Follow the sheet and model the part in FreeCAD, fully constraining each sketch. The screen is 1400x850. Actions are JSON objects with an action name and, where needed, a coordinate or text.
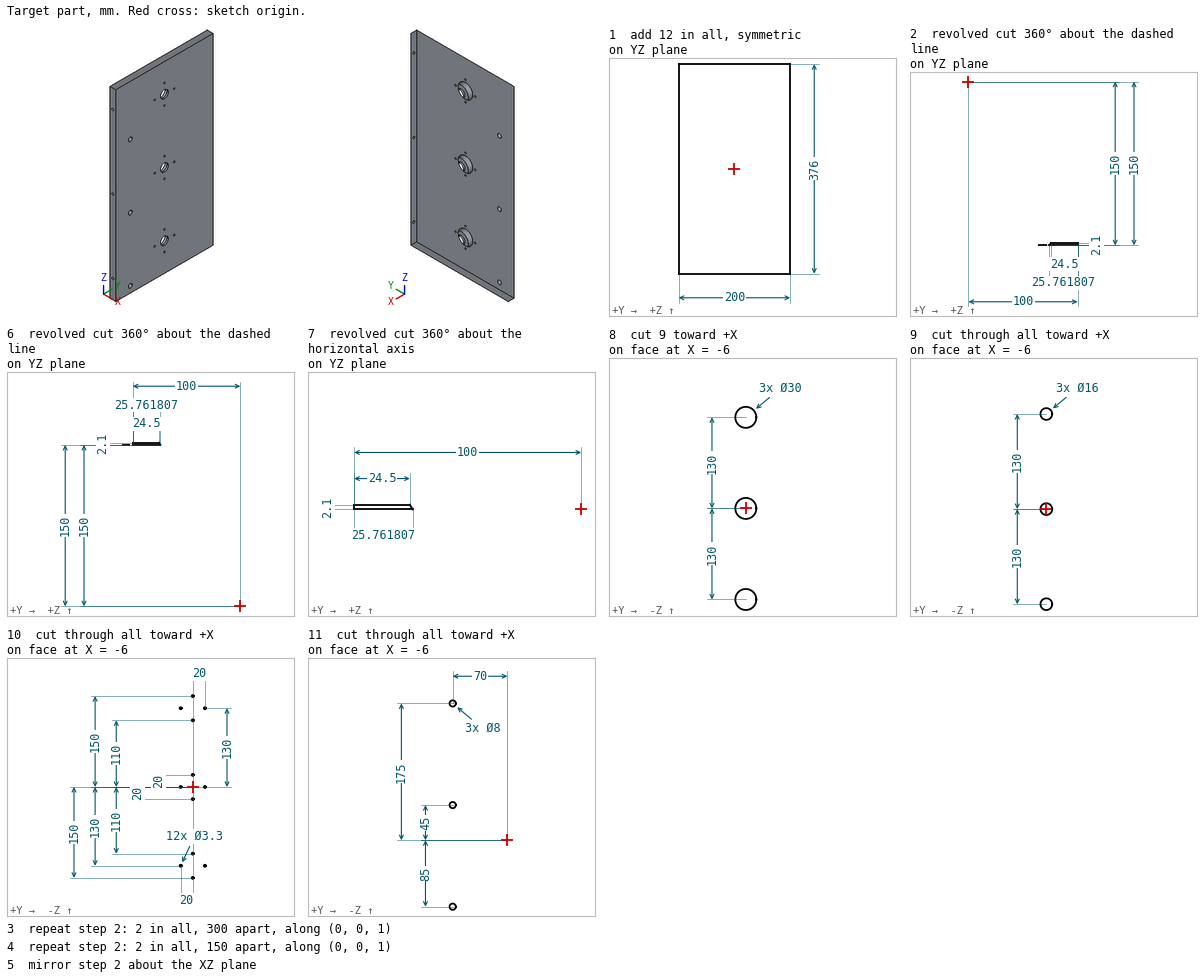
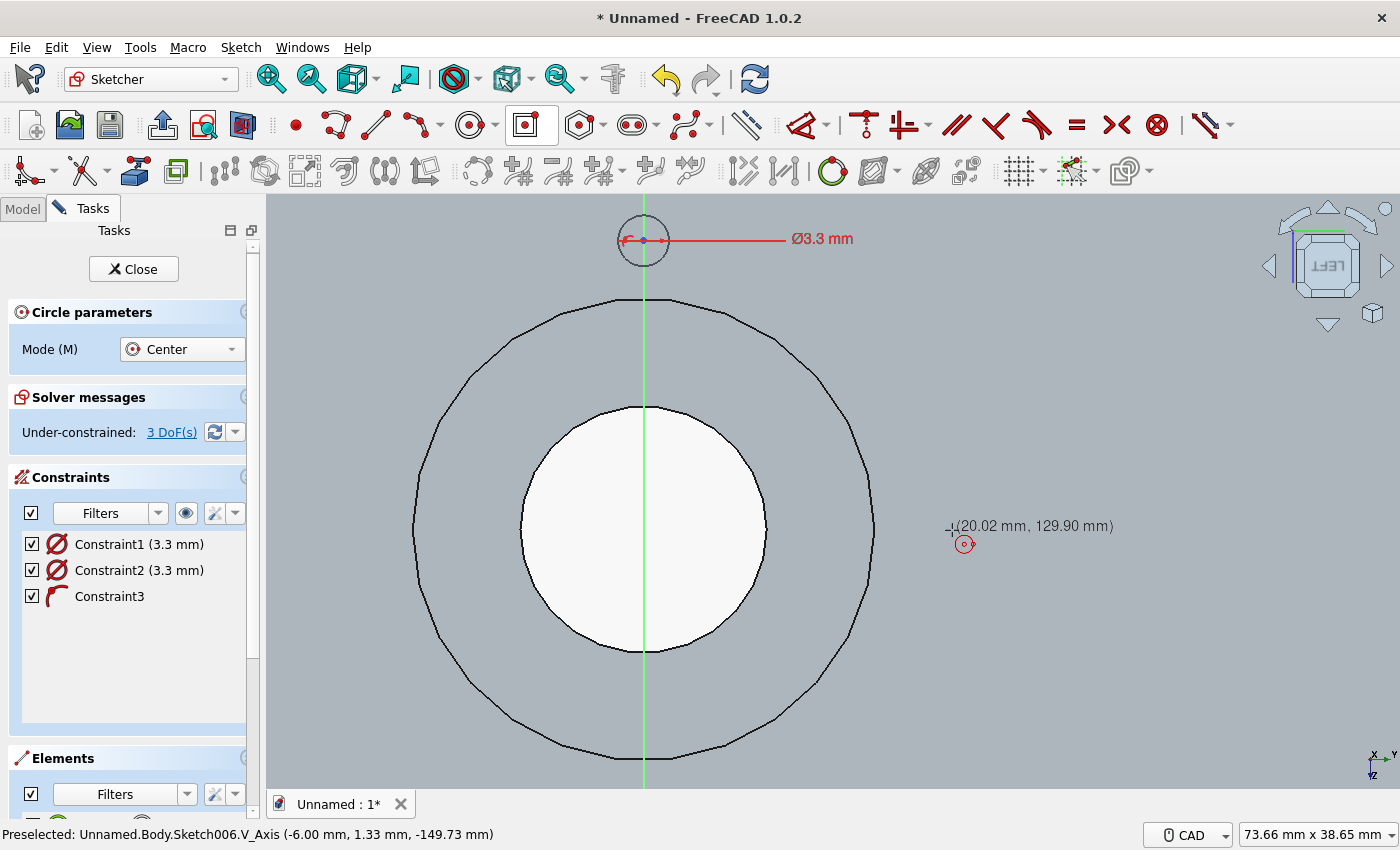
{"action": "scroll", "coordinate": [774, 328], "scroll_direction": "down", "scroll_amount": 13}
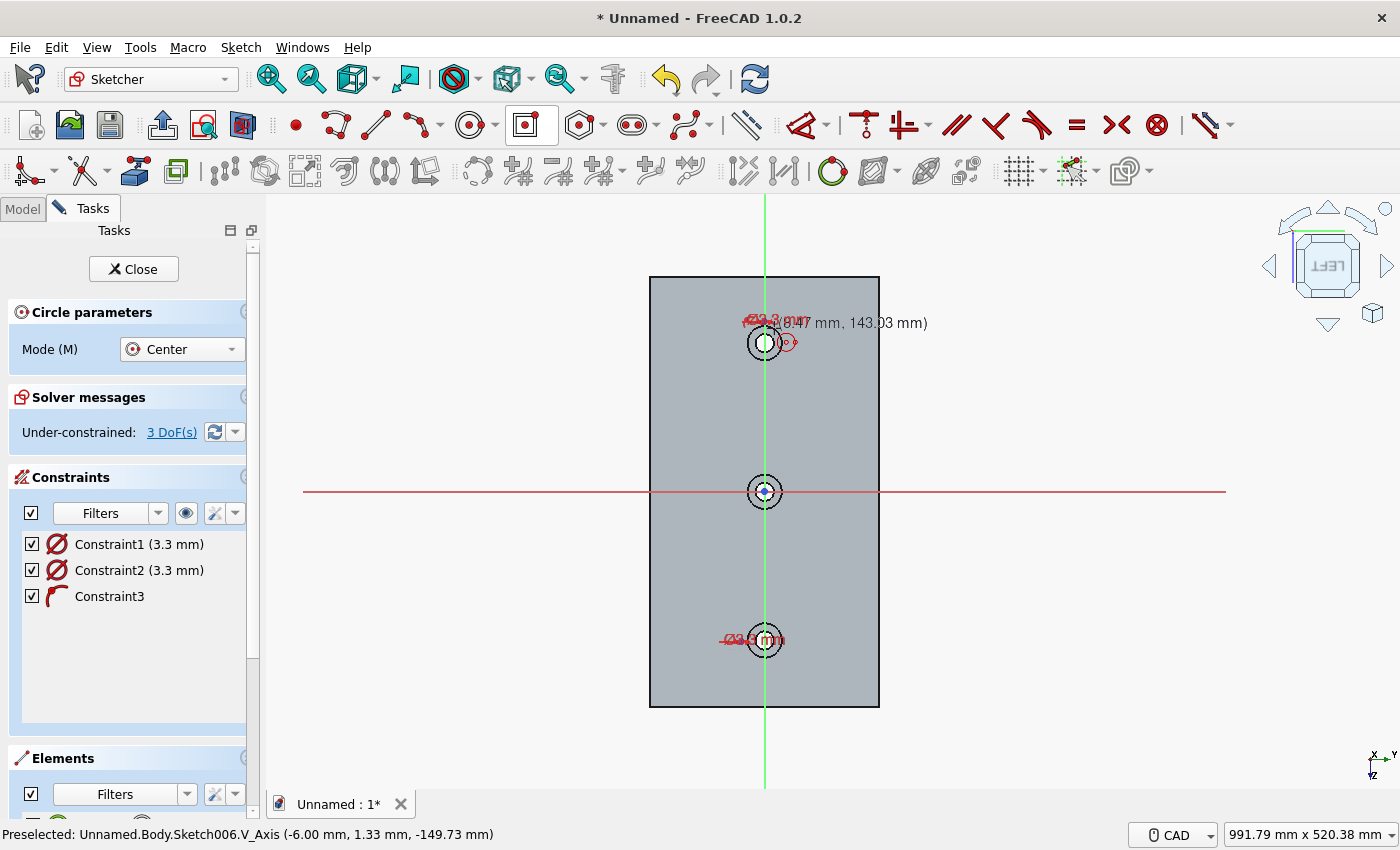
{"action": "left_click", "coordinate": [788, 343]}
{"action": "mouse_move", "coordinate": [789, 342]}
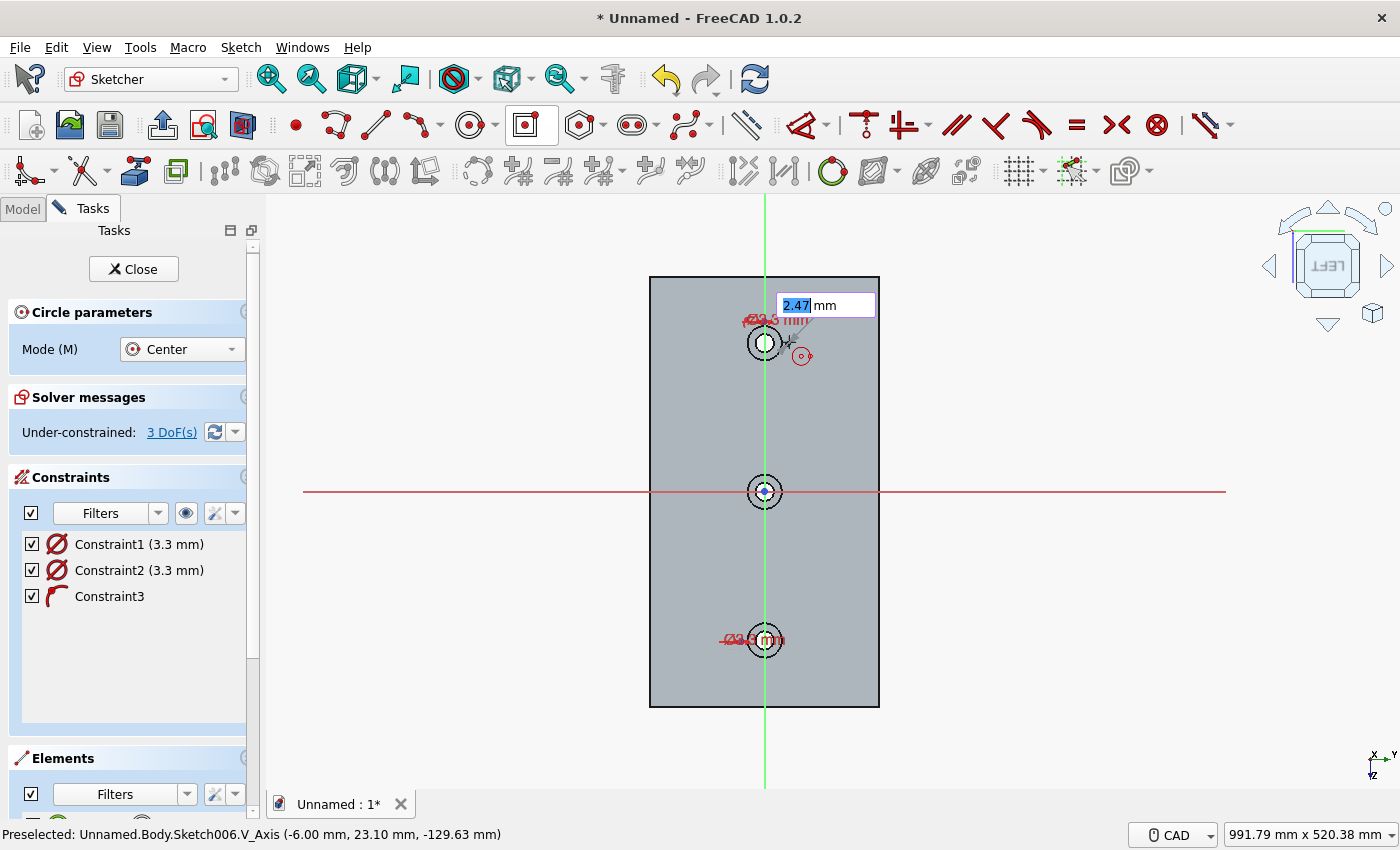
{"action": "type", "text": "3.3"}
{"action": "key", "text": "Return"}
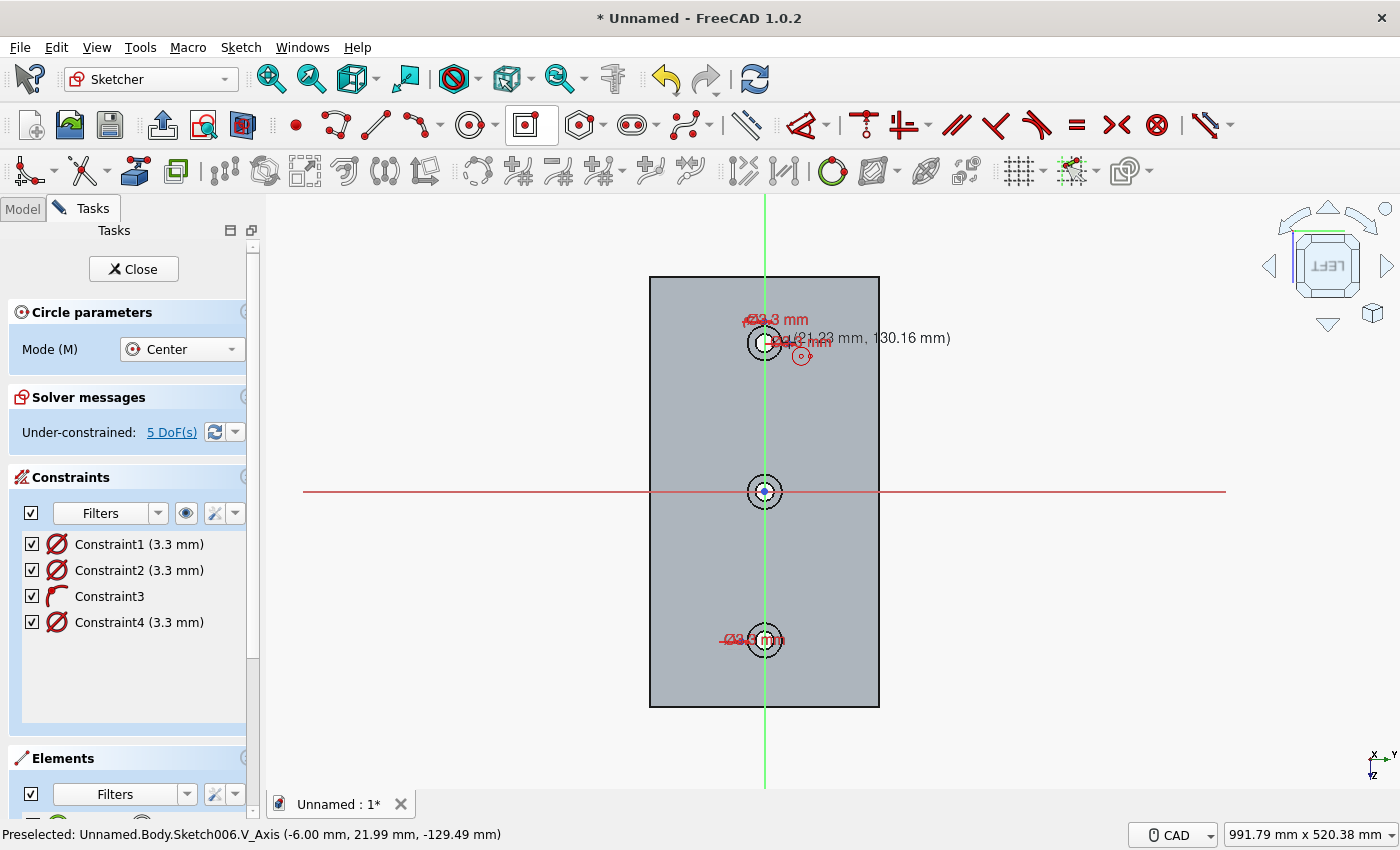
{"action": "scroll", "coordinate": [765, 366], "scroll_direction": "up", "scroll_amount": 13}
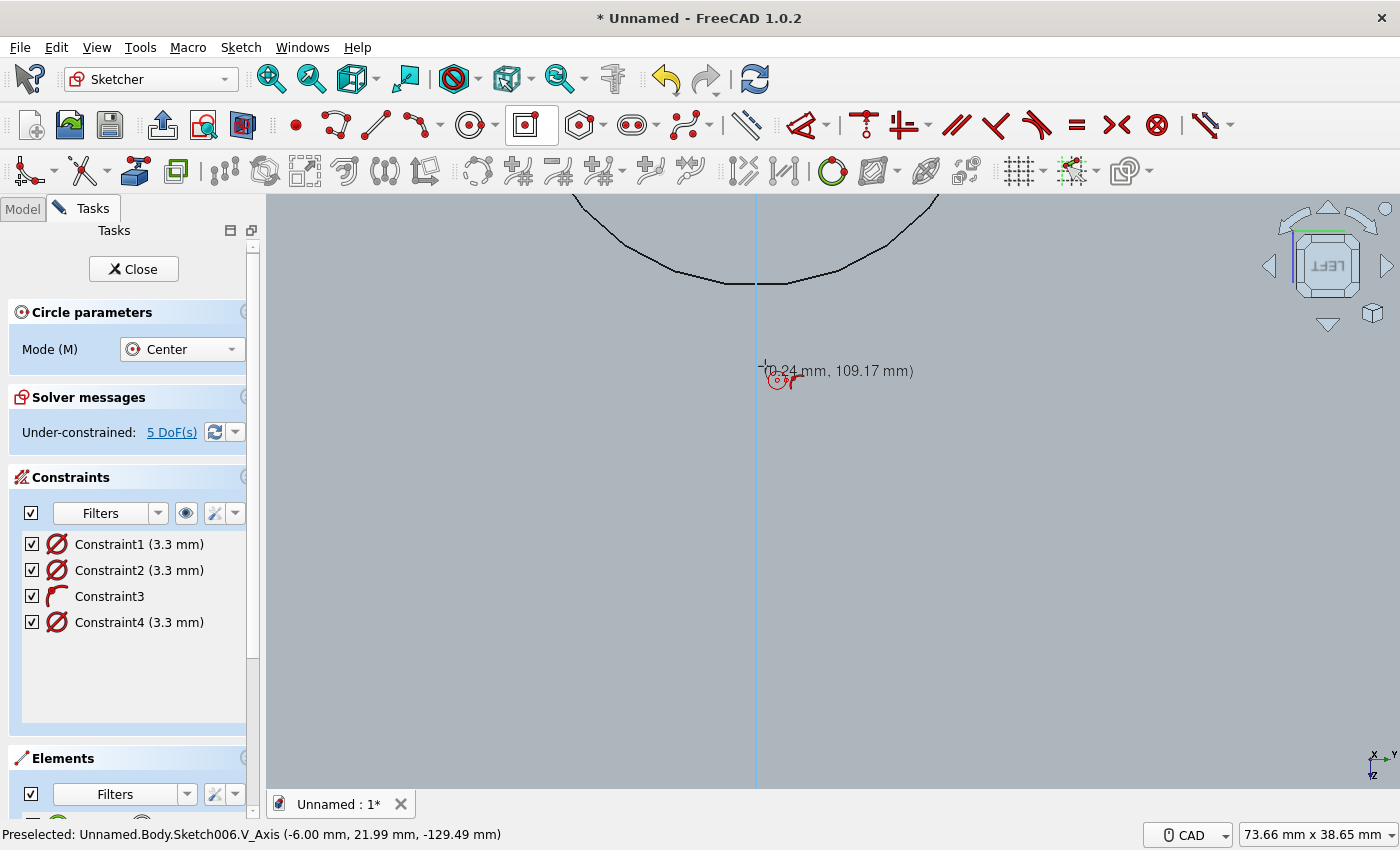
{"action": "scroll", "coordinate": [765, 366], "scroll_direction": "down", "scroll_amount": 13}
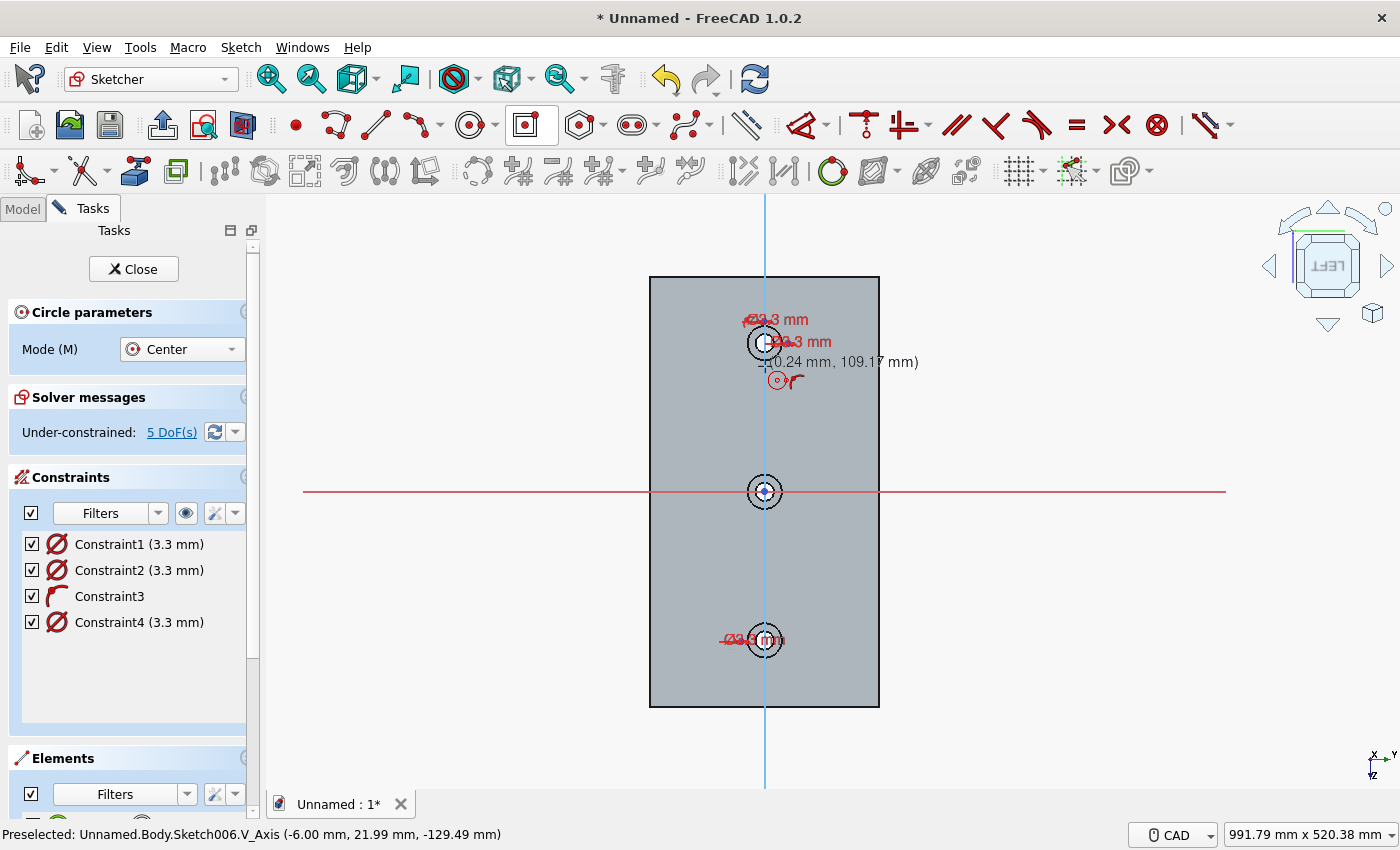
{"action": "left_click", "coordinate": [765, 366]}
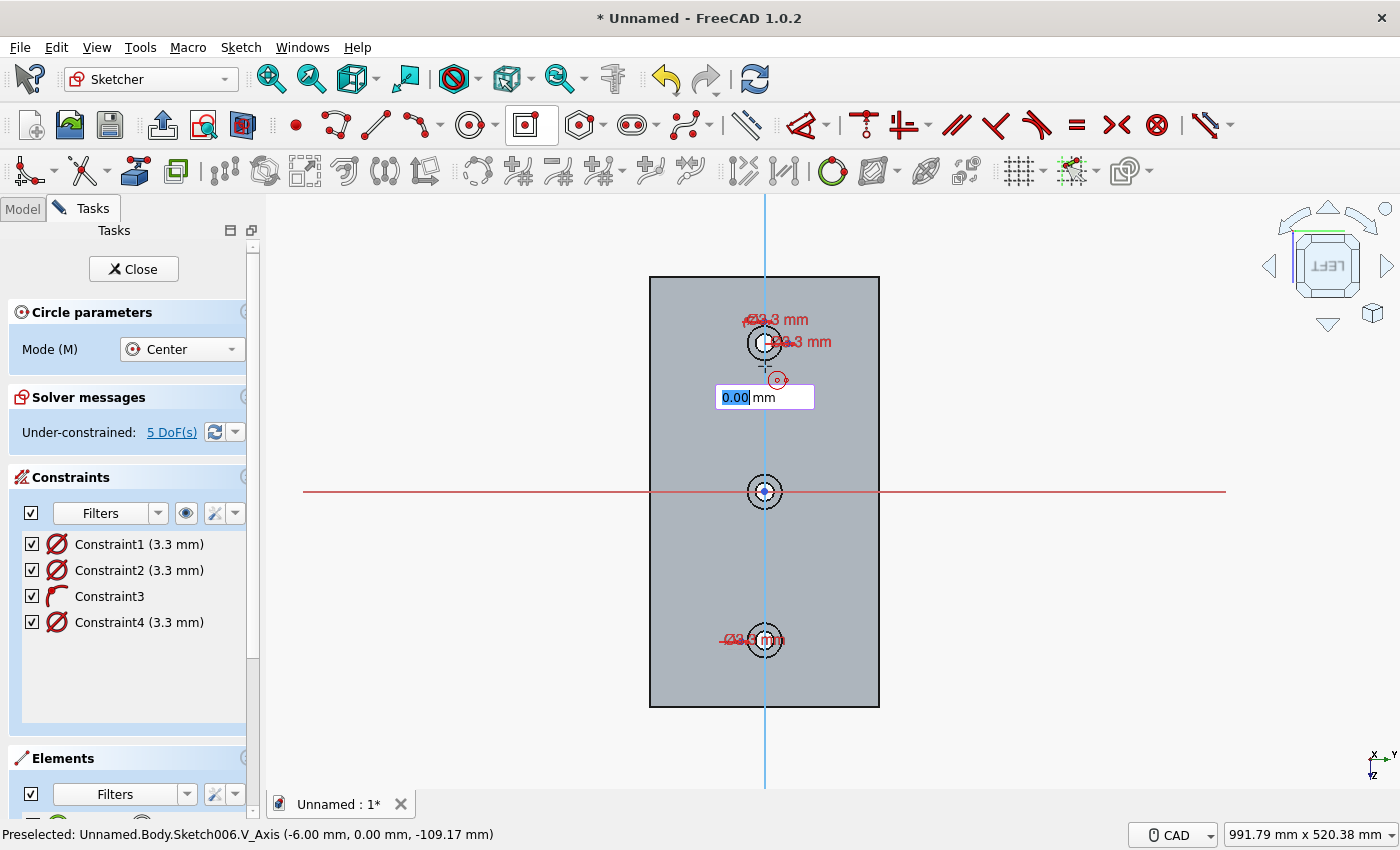
{"action": "scroll", "coordinate": [767, 365], "scroll_direction": "up", "scroll_amount": 11}
{"action": "mouse_move", "coordinate": [759, 366]}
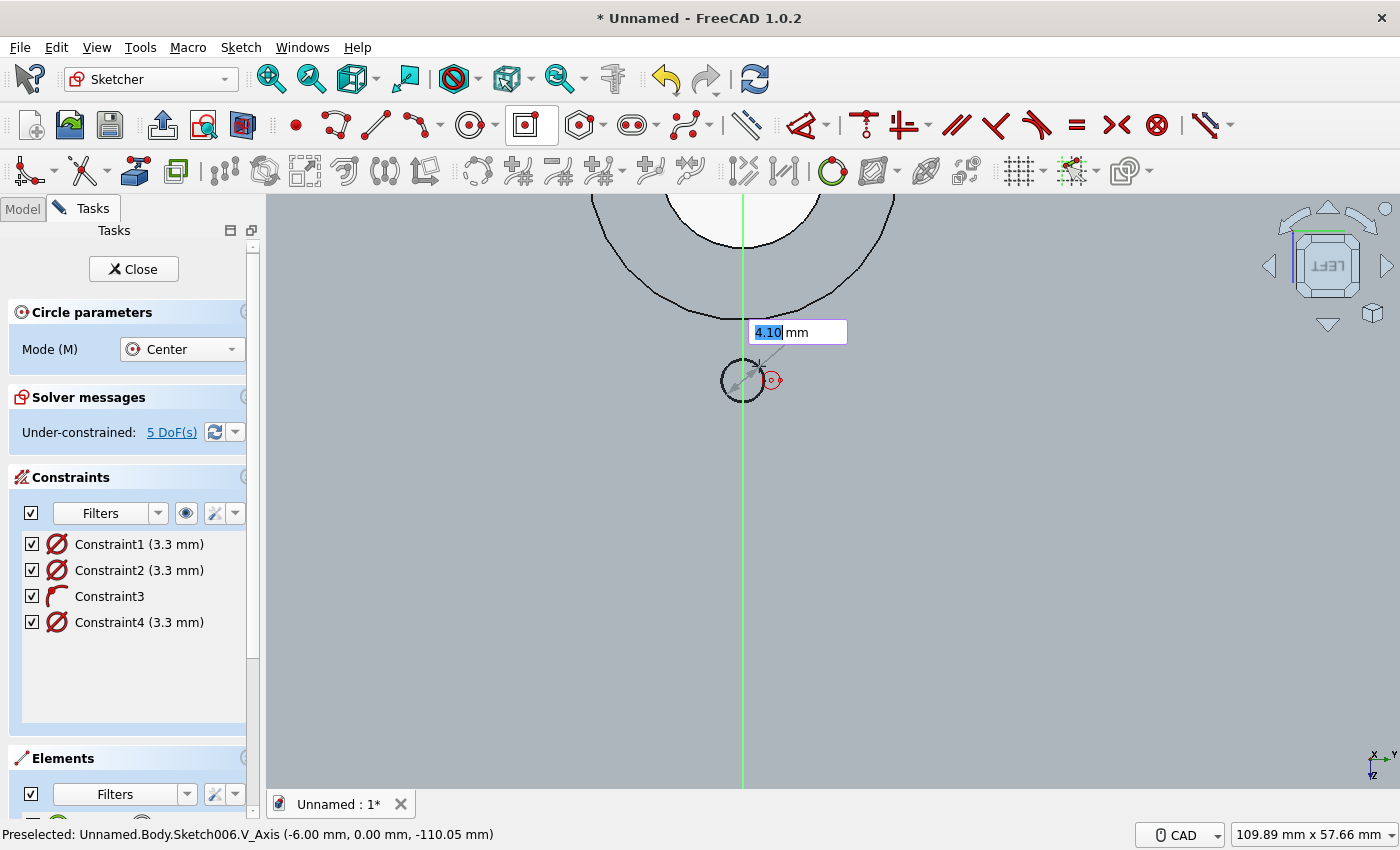
{"action": "type", "text": "3.3"}
{"action": "key", "text": "Return"}